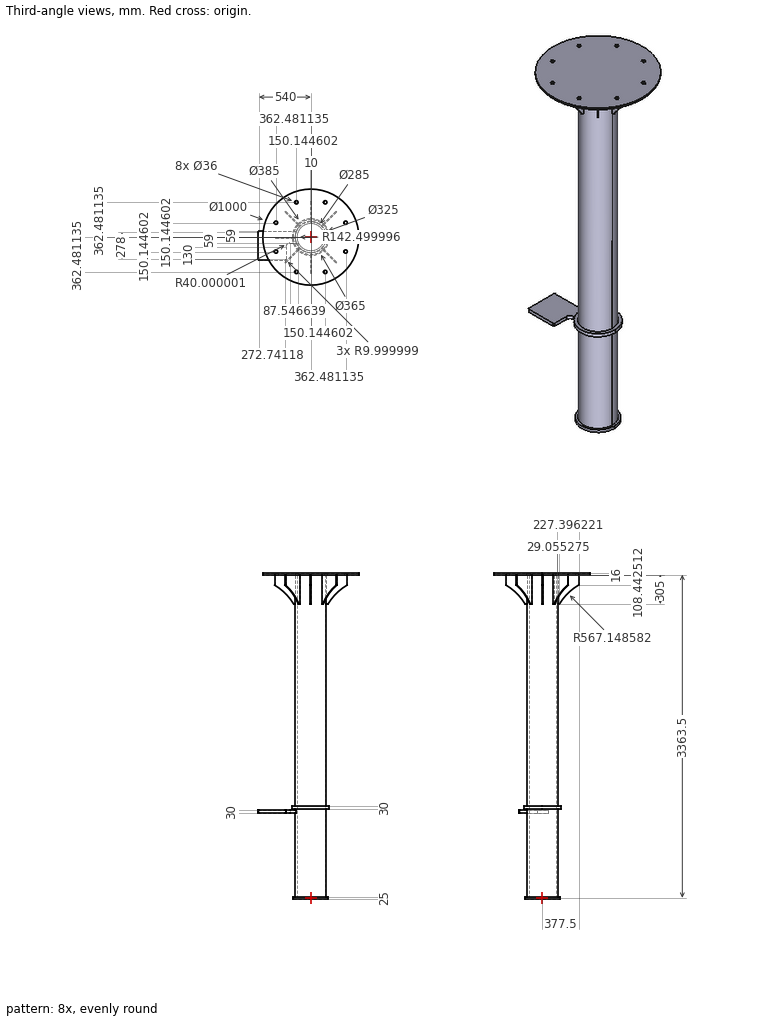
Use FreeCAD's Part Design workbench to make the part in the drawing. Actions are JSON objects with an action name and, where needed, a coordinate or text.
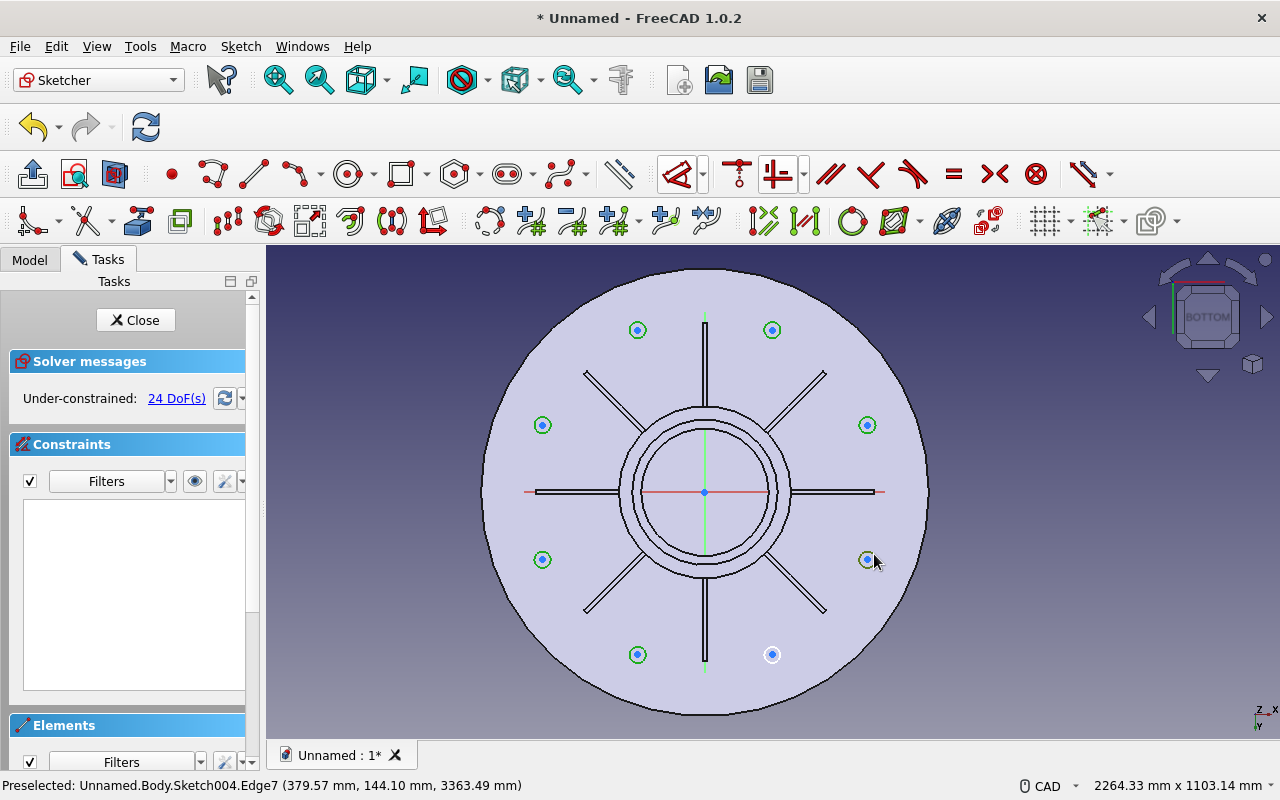
{"action": "scroll", "coordinate": [778, 649], "scroll_direction": "up", "scroll_amount": 3}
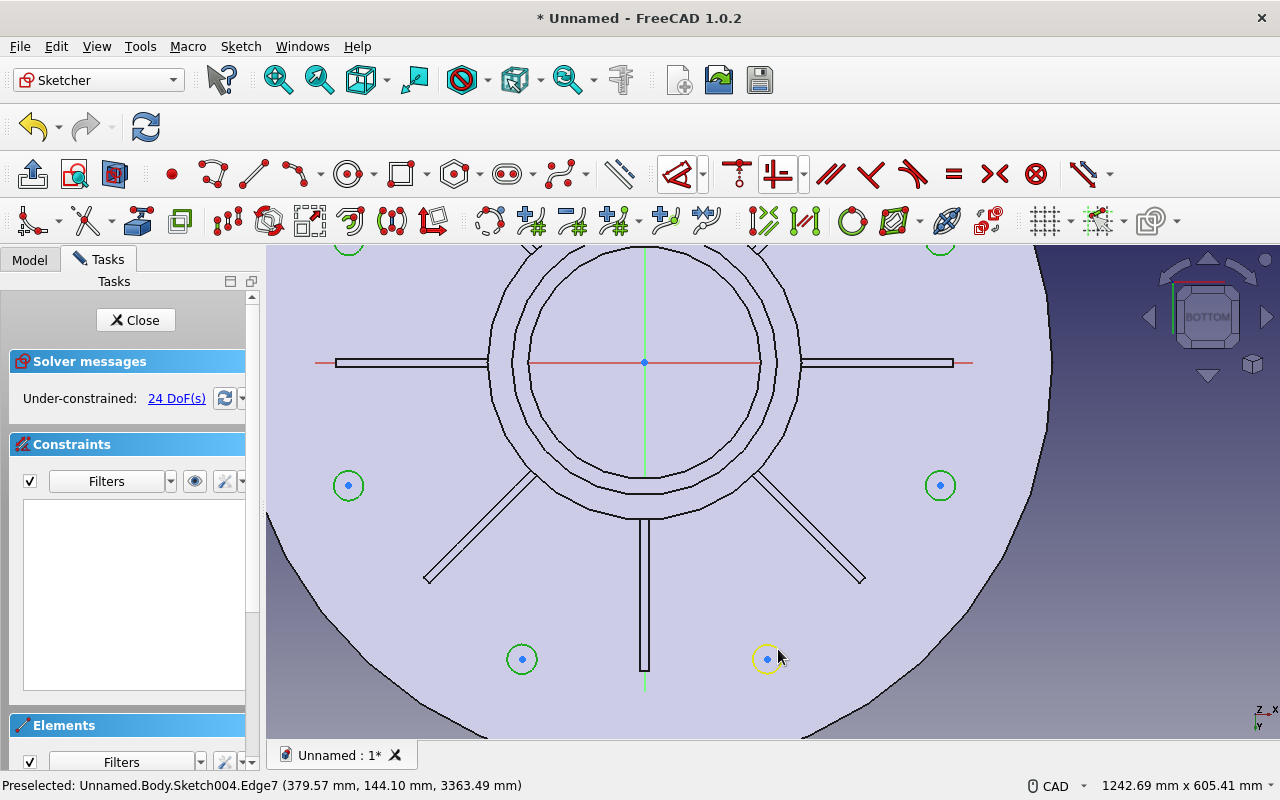
{"action": "left_click", "coordinate": [777, 649]}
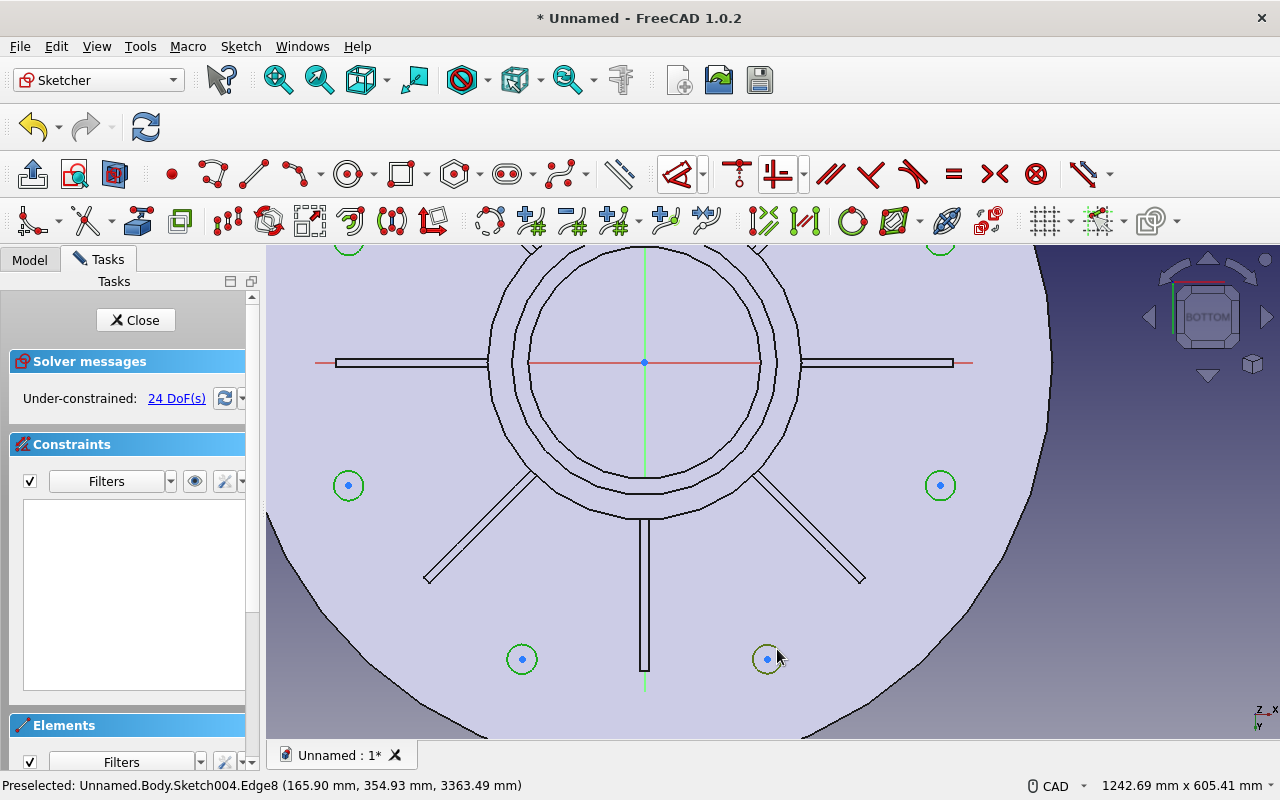
{"action": "key", "text": "e"}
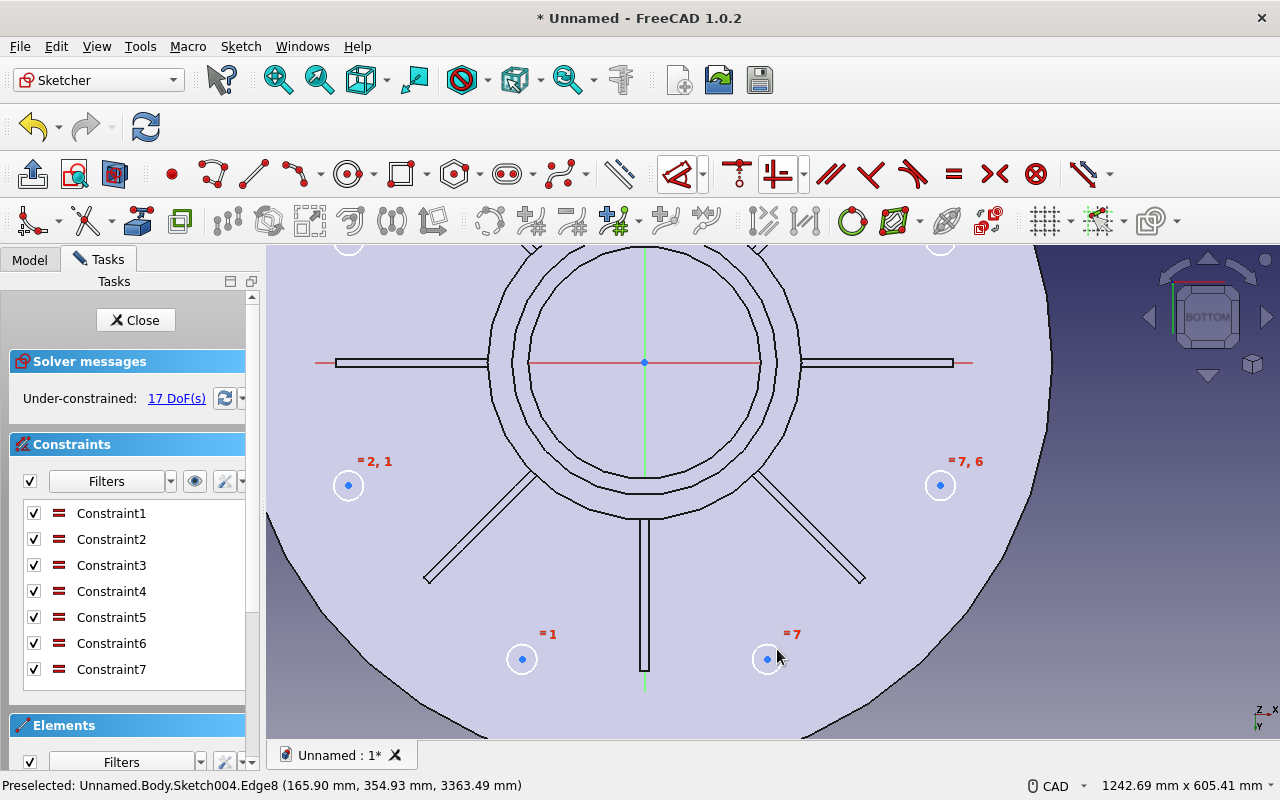
{"action": "left_click", "coordinate": [349, 486]}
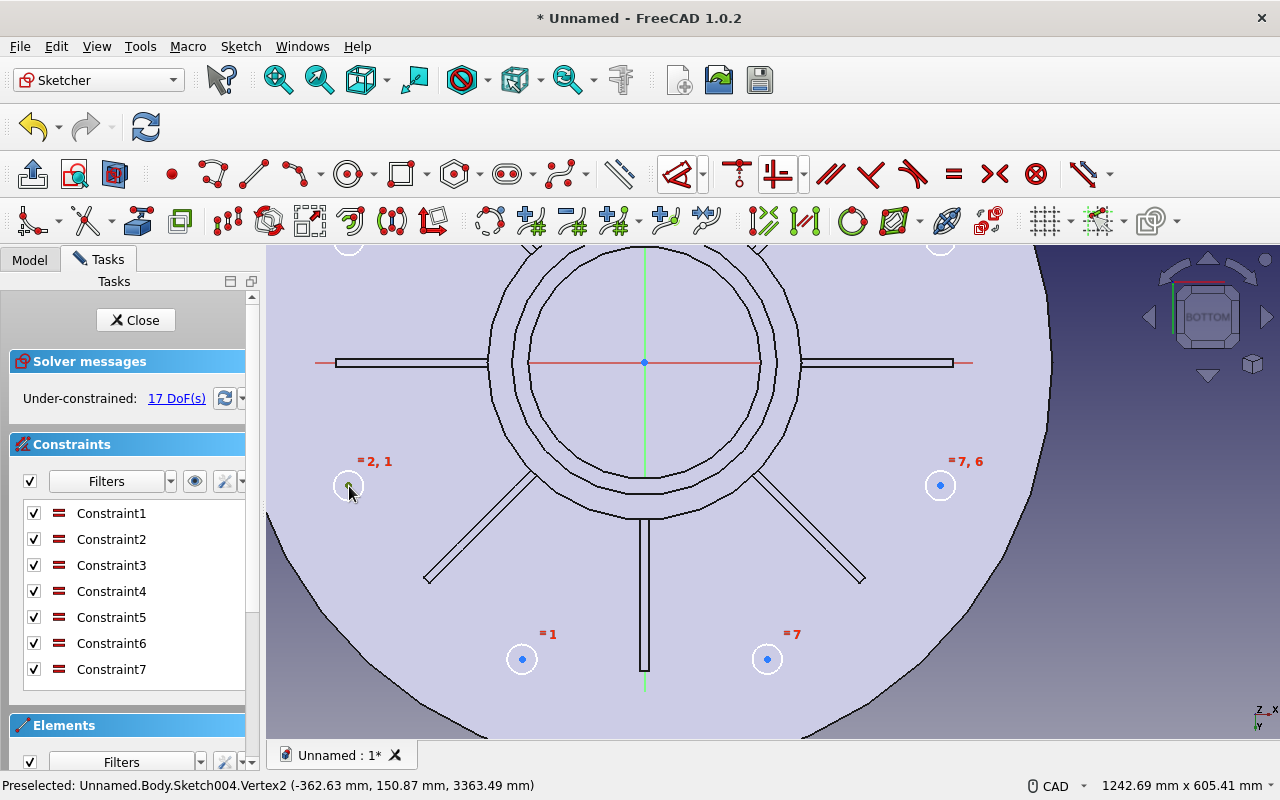
{"action": "scroll", "coordinate": [777, 649], "scroll_direction": "down", "scroll_amount": 3}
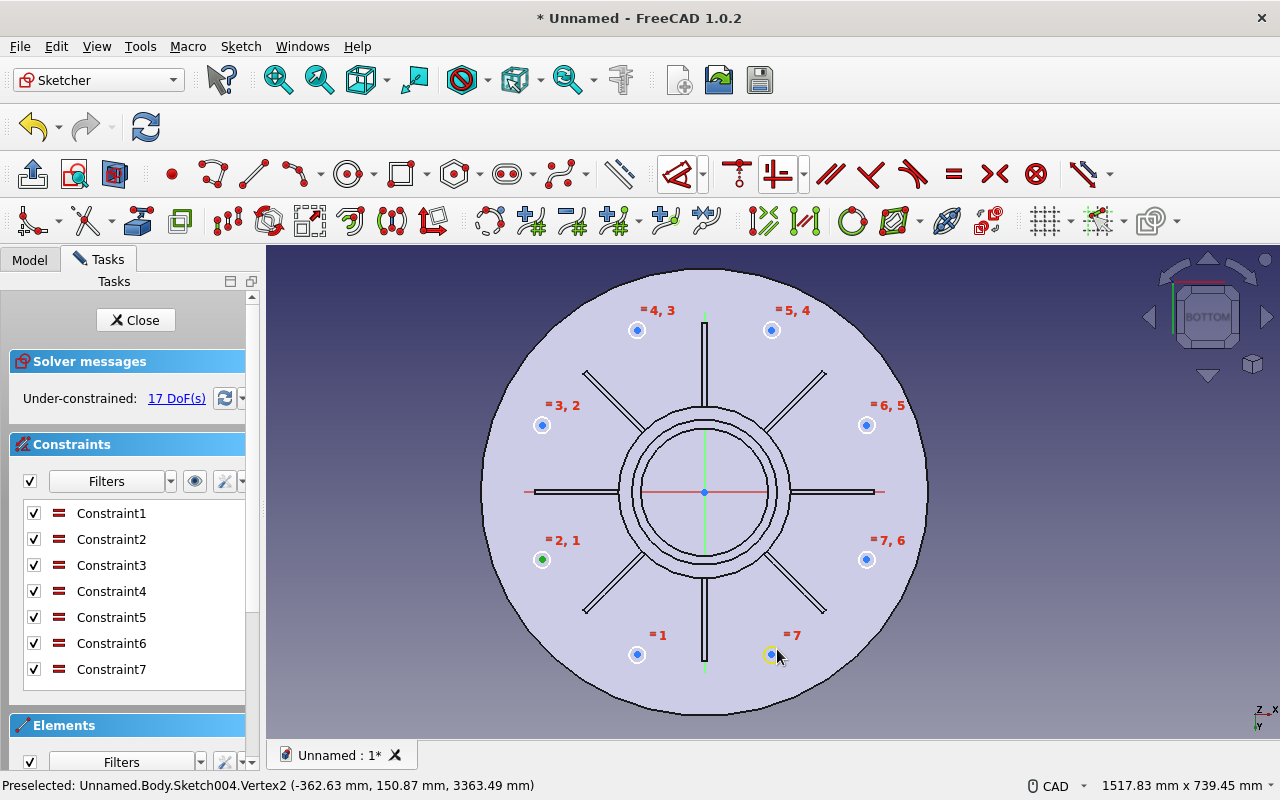
{"action": "left_click", "coordinate": [542, 425]}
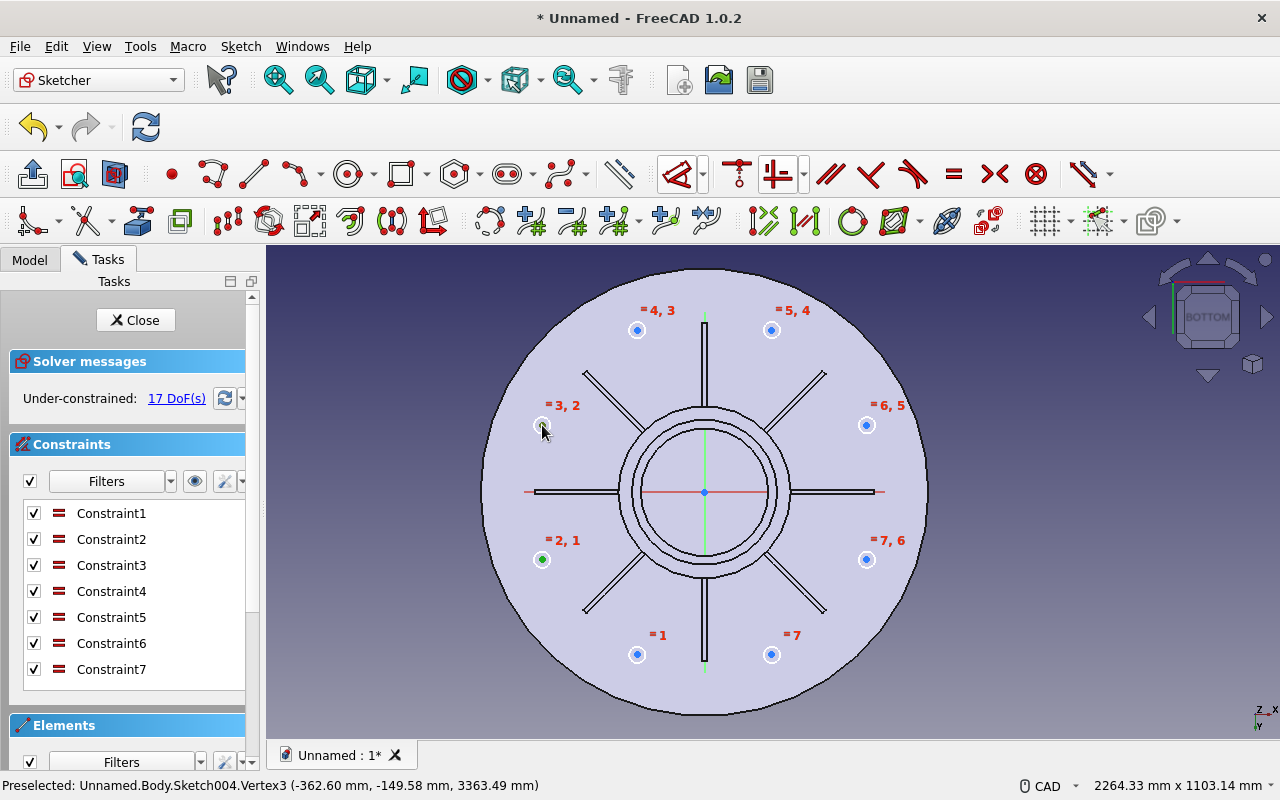
{"action": "key", "text": "v"}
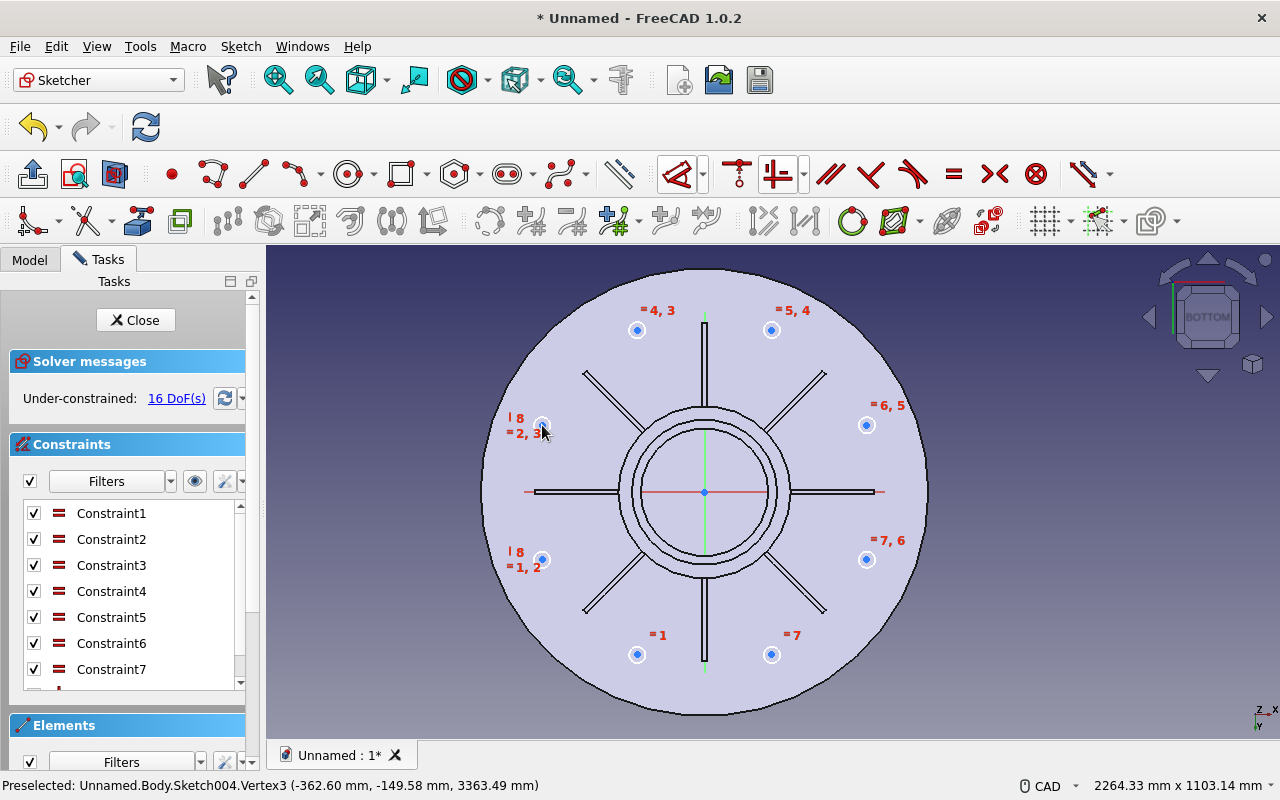
{"action": "left_click", "coordinate": [637, 655]}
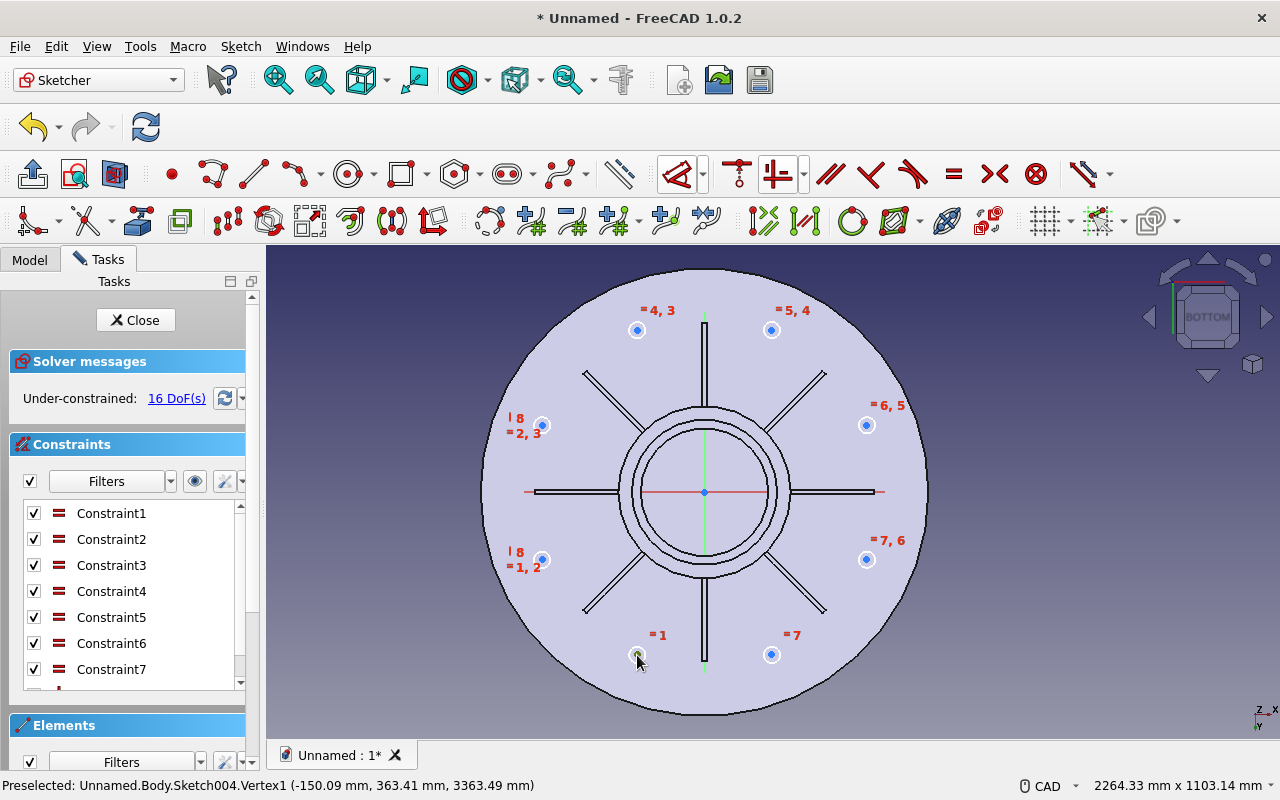
{"action": "left_click", "coordinate": [637, 330]}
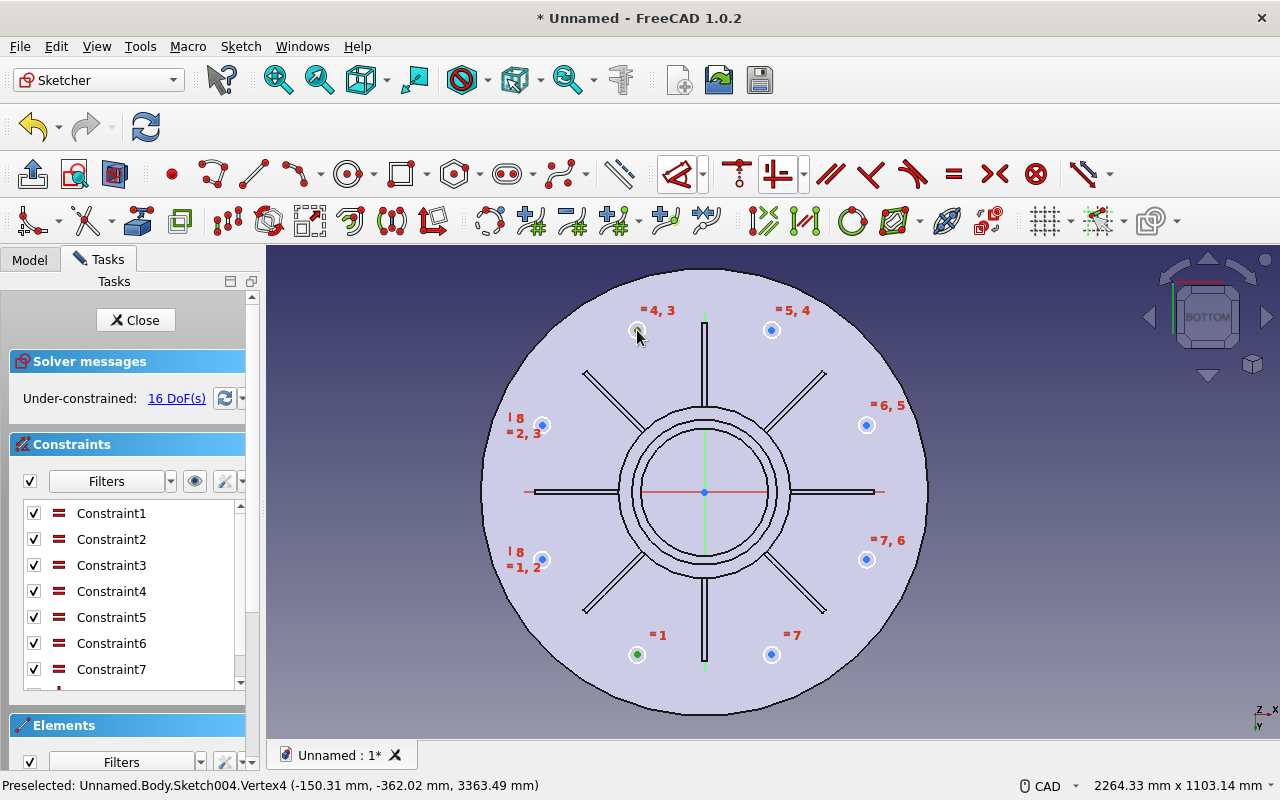
{"action": "key", "text": "v"}